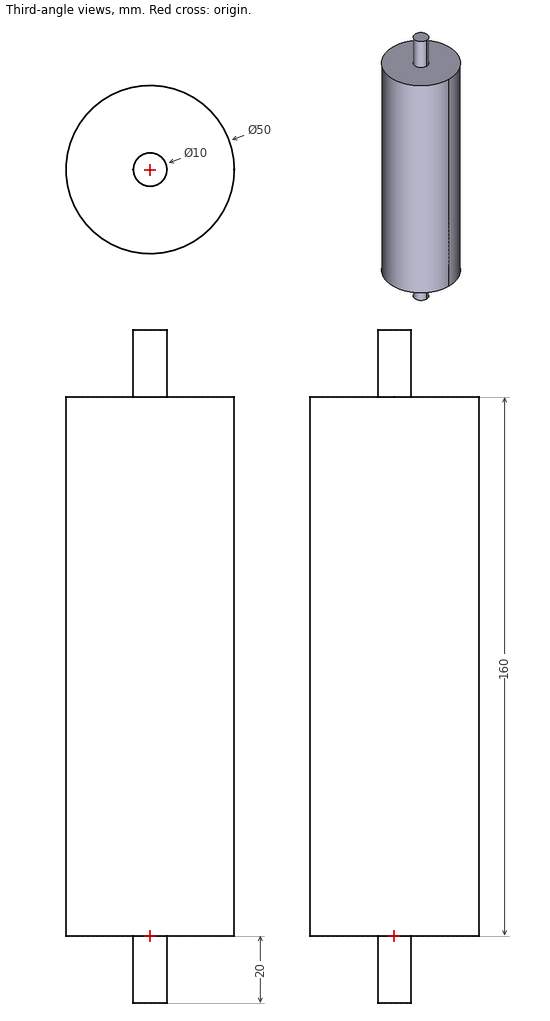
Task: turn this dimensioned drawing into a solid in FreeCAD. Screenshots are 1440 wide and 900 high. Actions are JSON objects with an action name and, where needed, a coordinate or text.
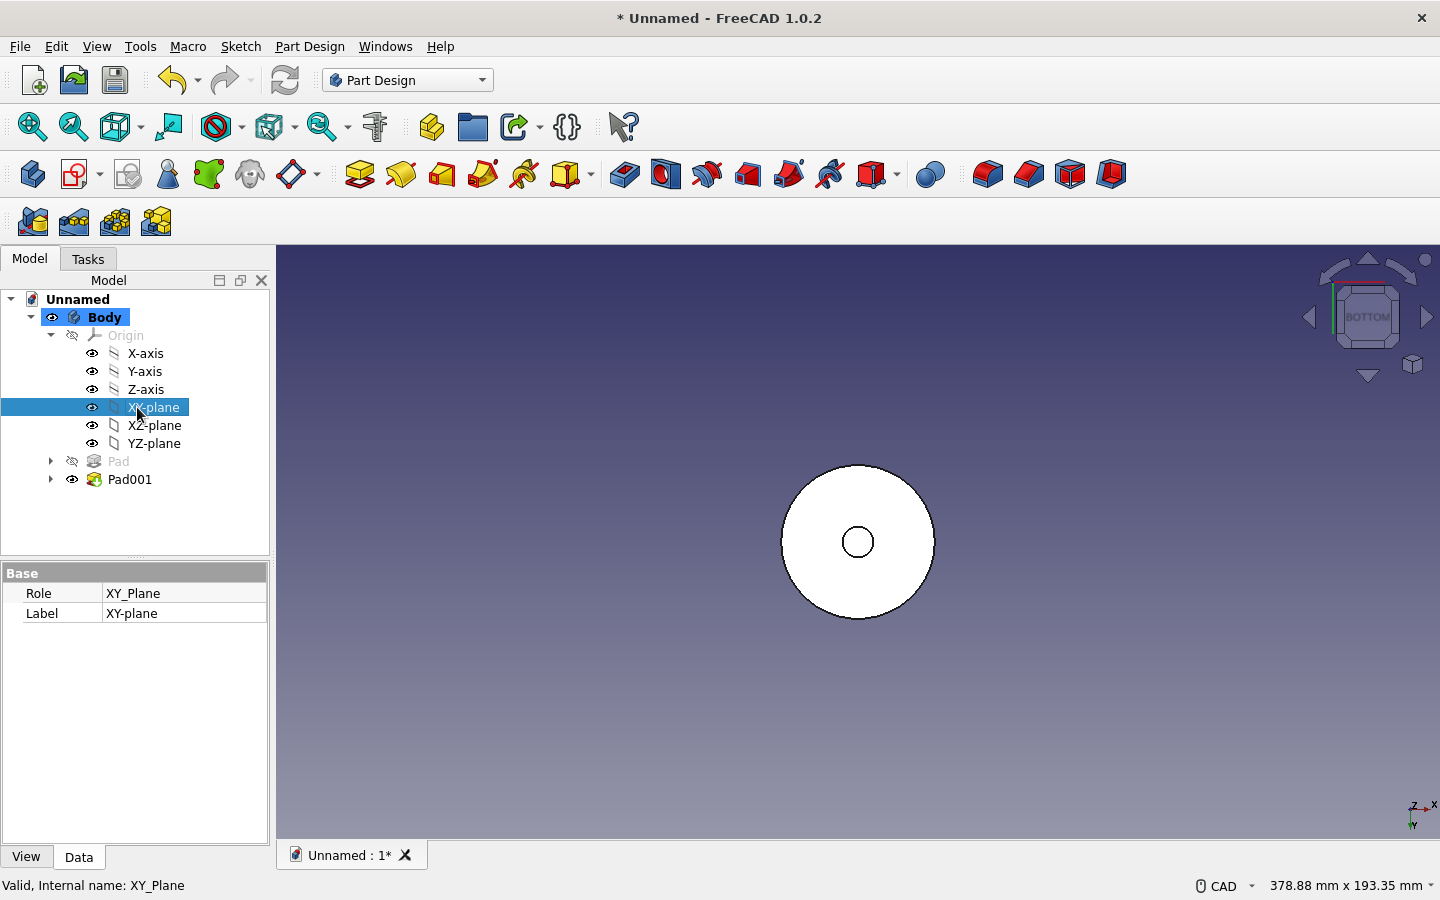
{"action": "left_click", "coordinate": [290, 174]}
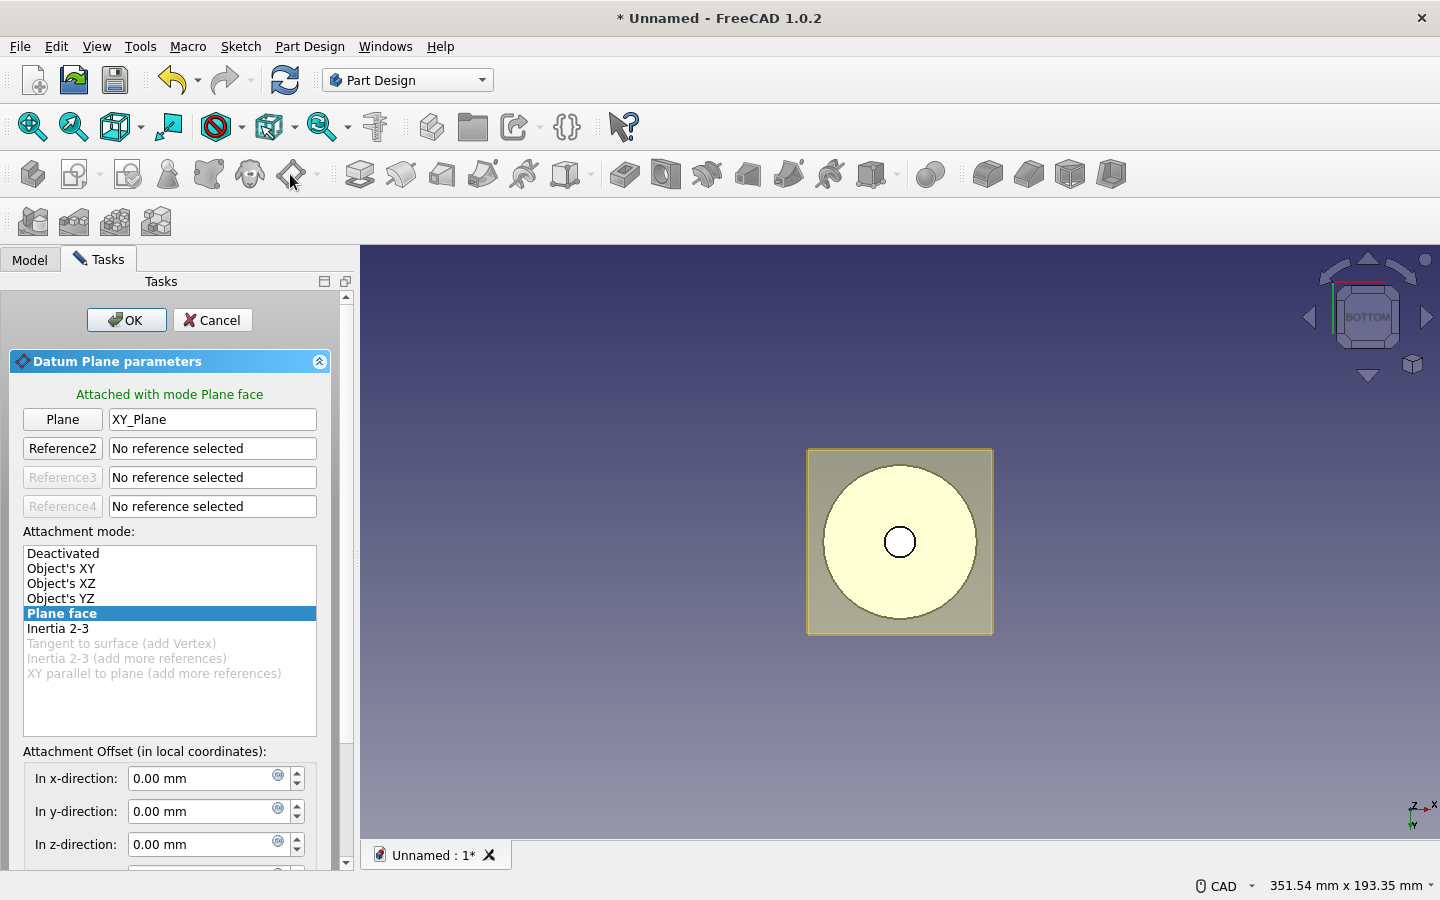
{"action": "triple_click", "coordinate": [210, 844]}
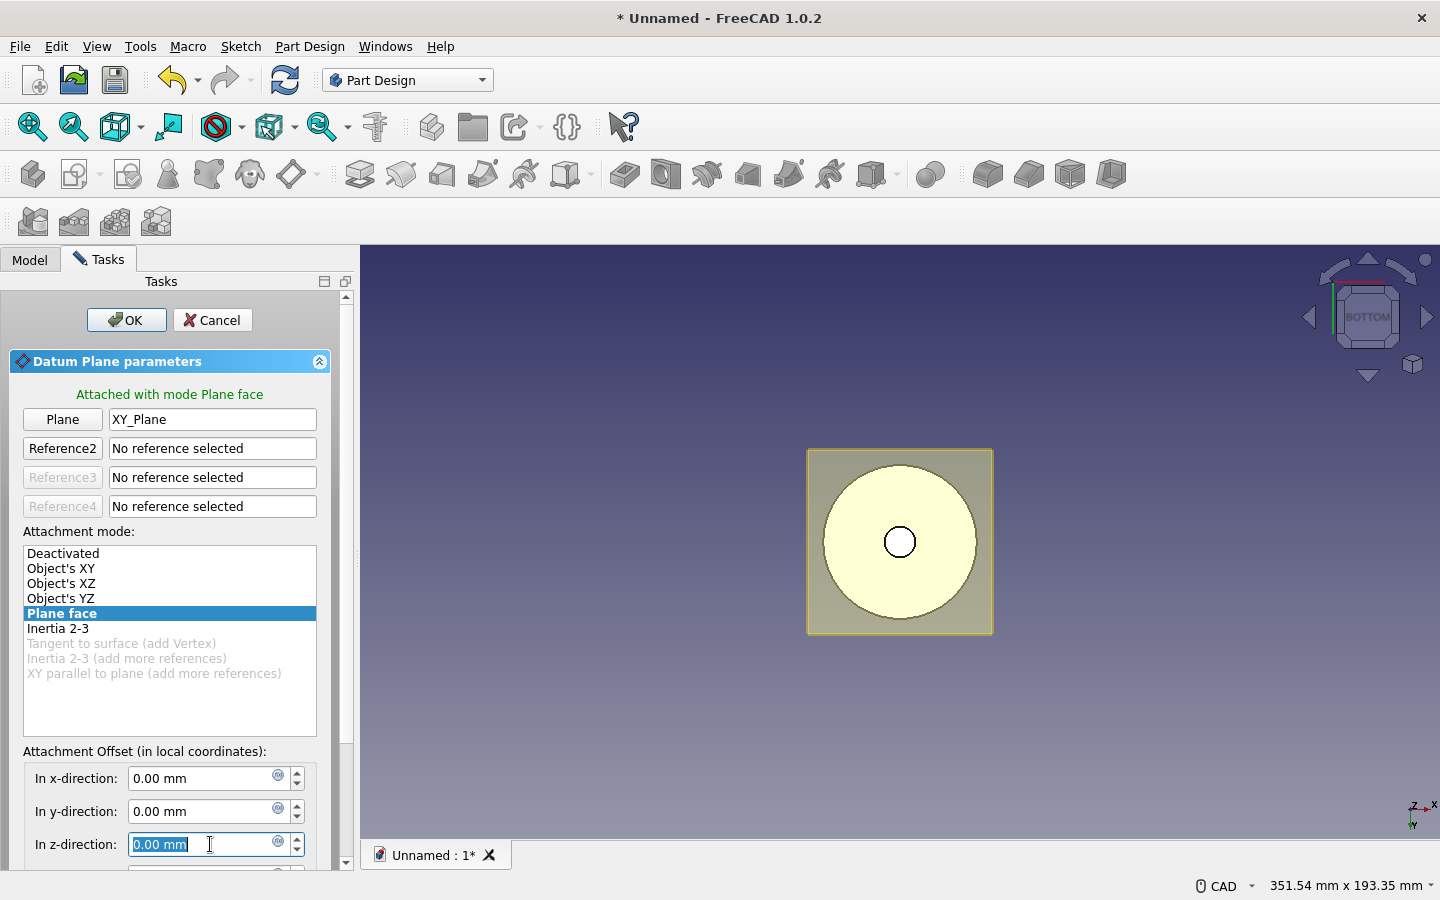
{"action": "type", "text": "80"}
{"action": "key", "text": "Tab"}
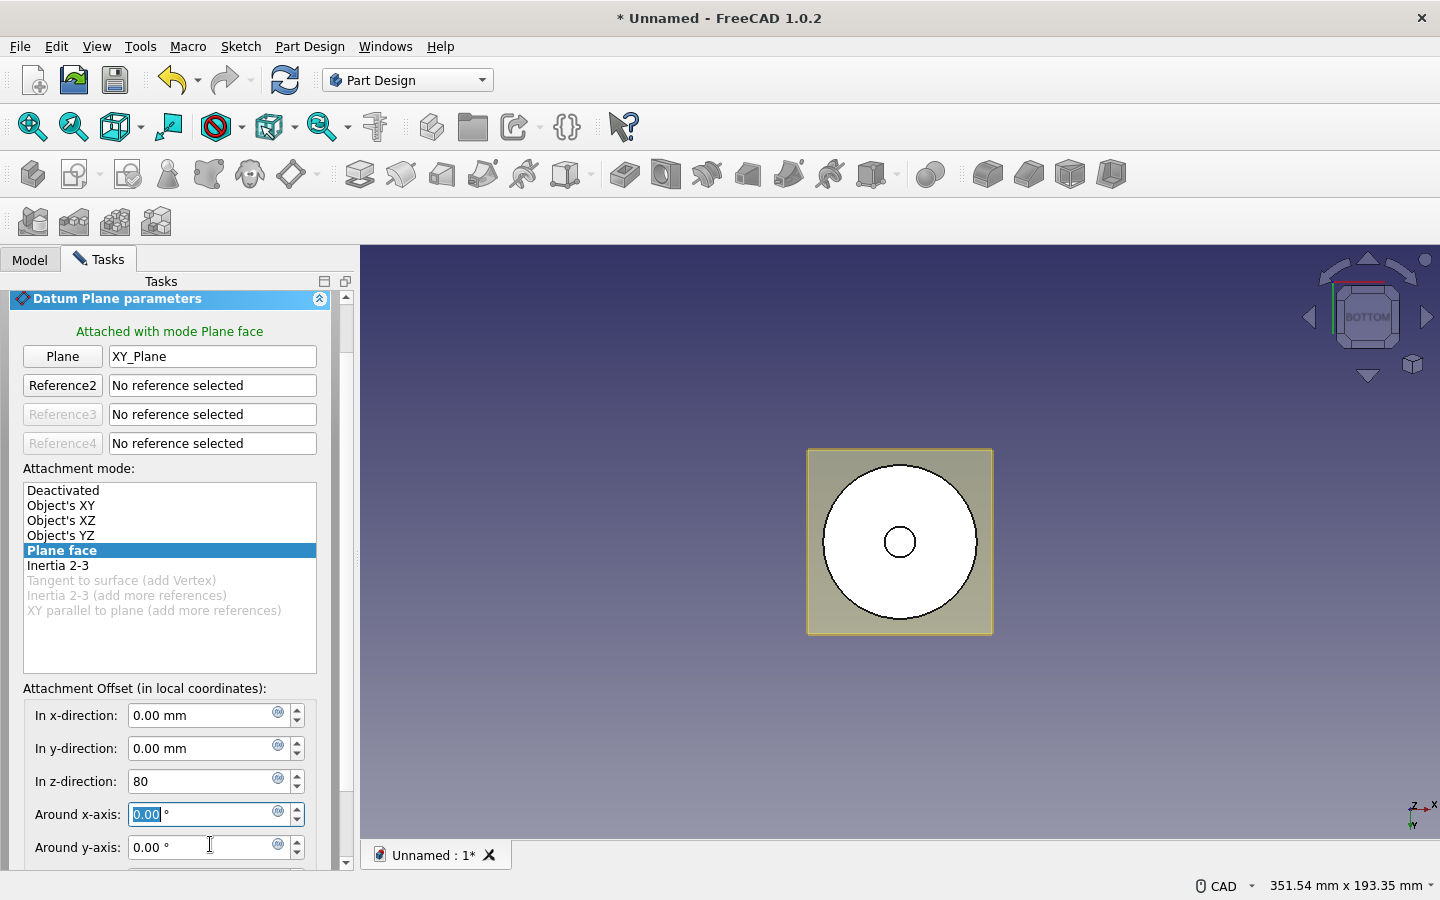
{"action": "scroll", "coordinate": [346, 580], "scroll_direction": "up", "scroll_amount": 2}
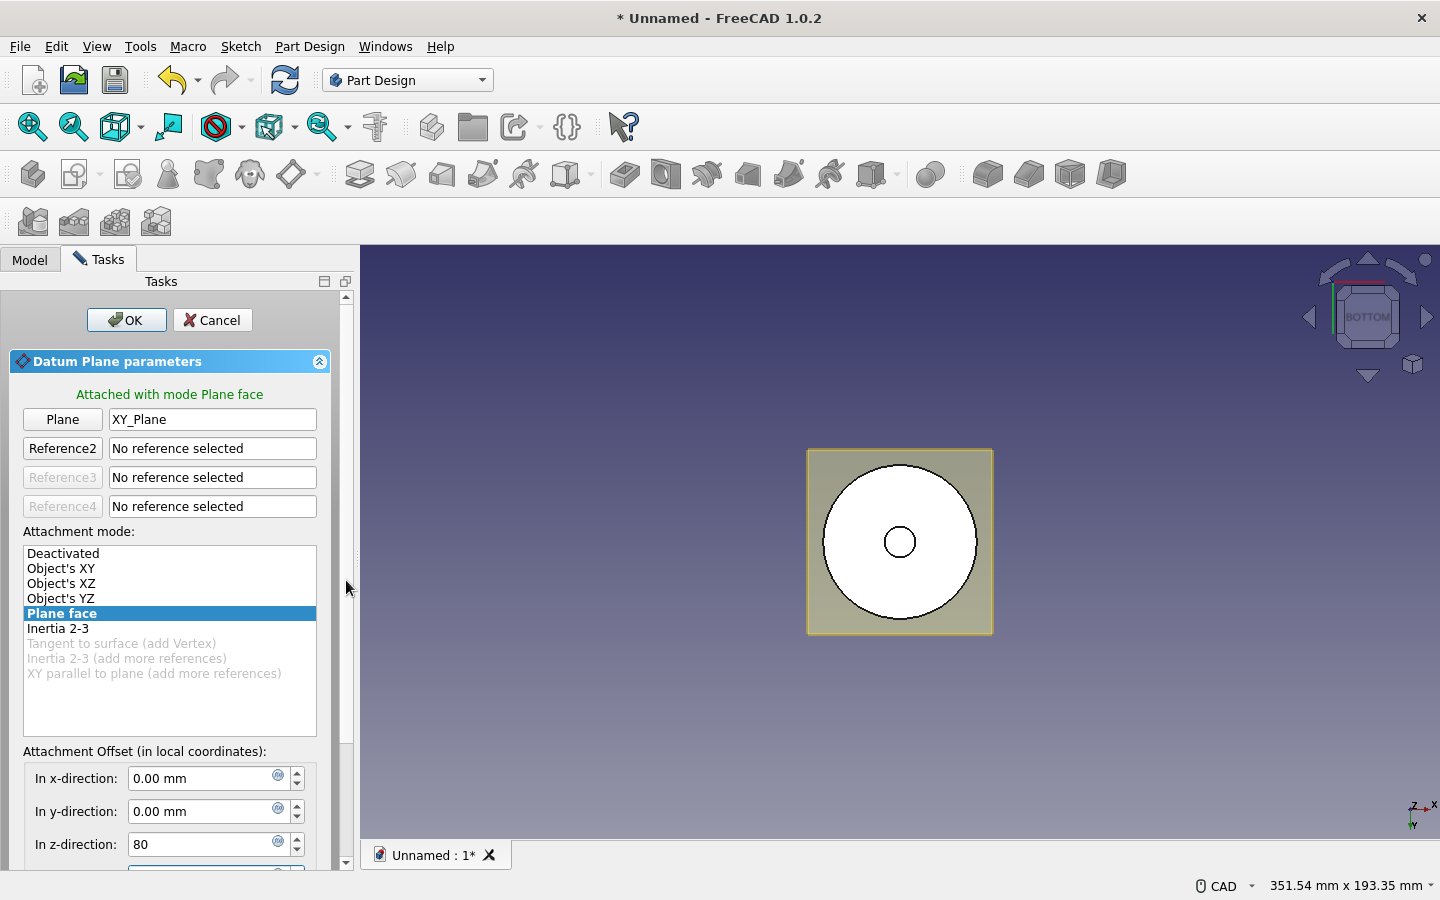
{"action": "left_click", "coordinate": [127, 320]}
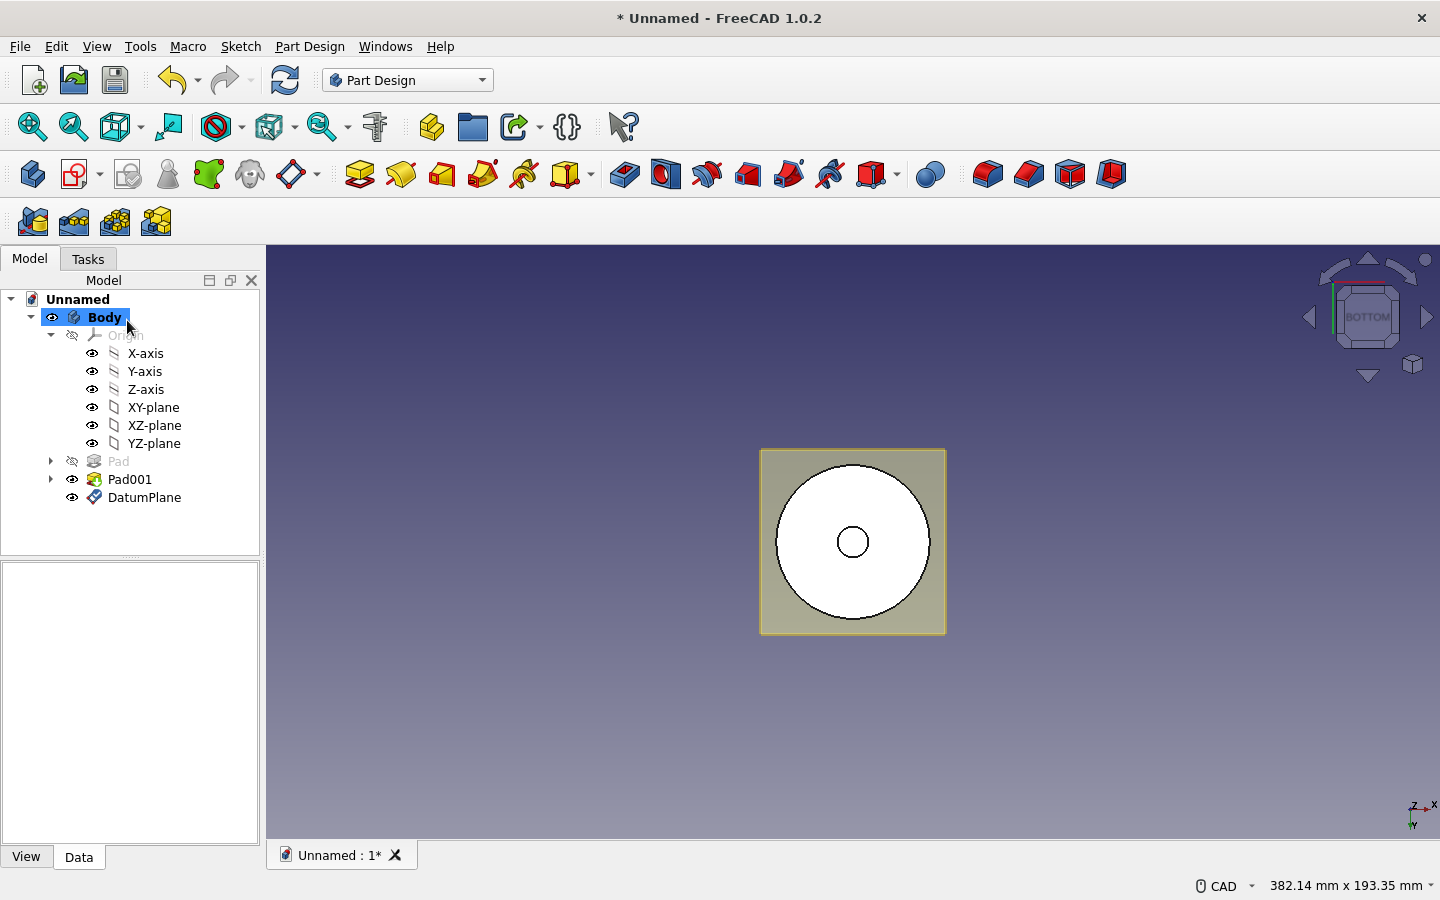
{"action": "left_click", "coordinate": [117, 479]}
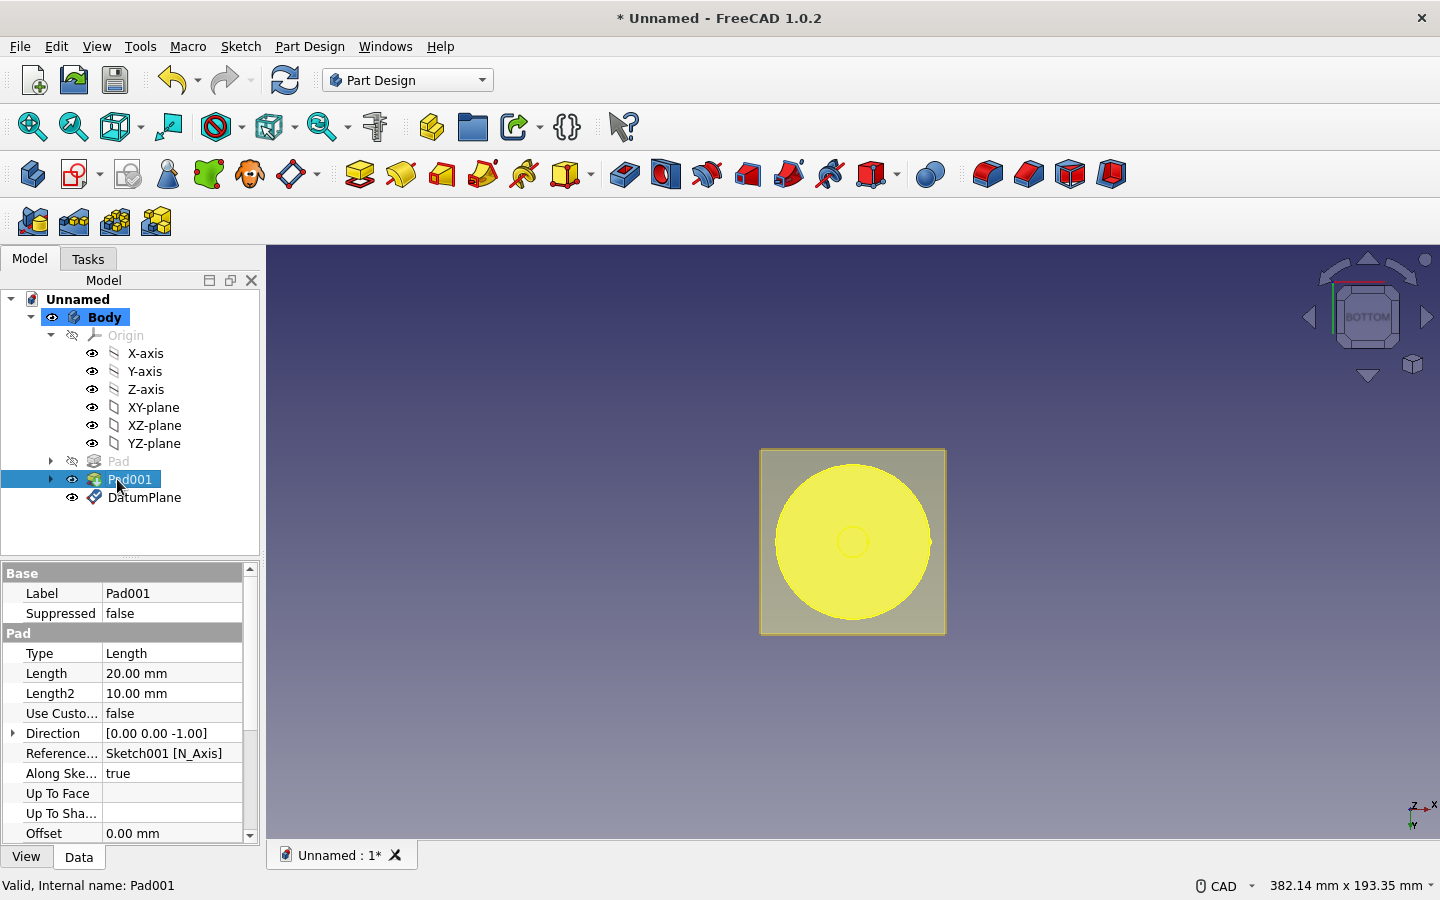
{"action": "left_click", "coordinate": [33, 222]}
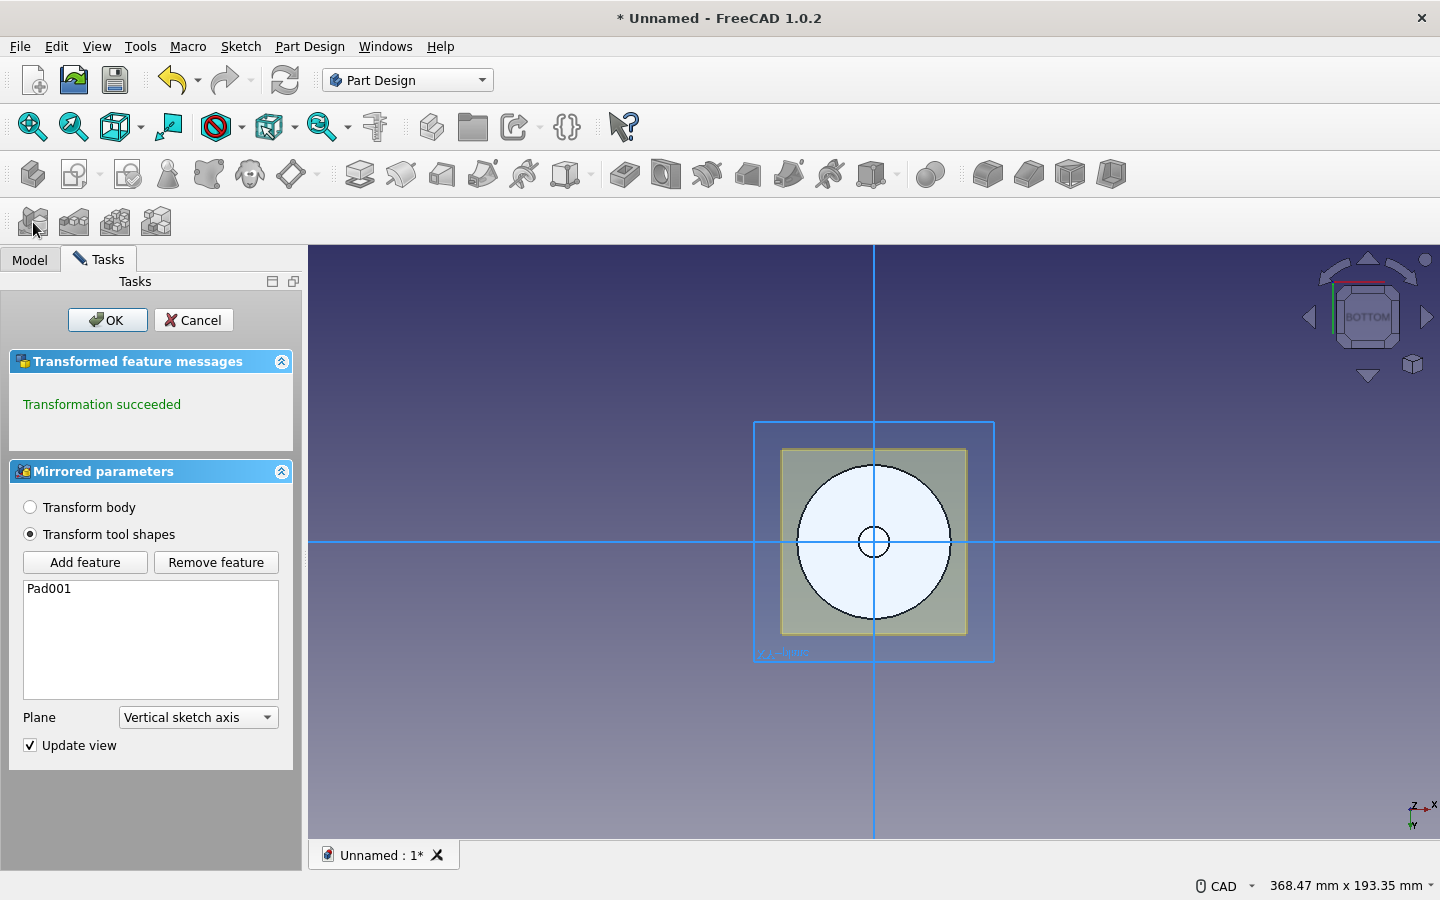
{"action": "left_click", "coordinate": [199, 718]}